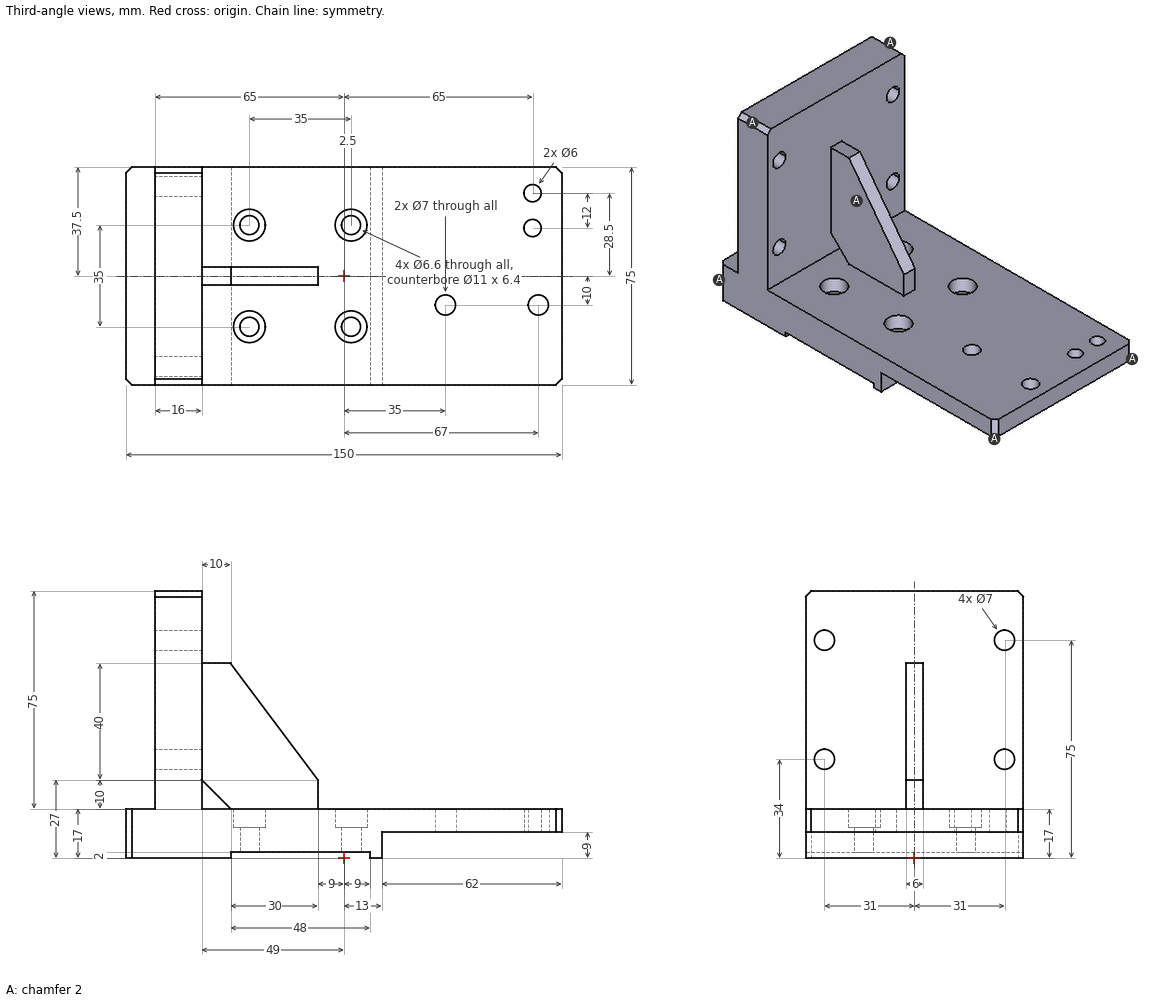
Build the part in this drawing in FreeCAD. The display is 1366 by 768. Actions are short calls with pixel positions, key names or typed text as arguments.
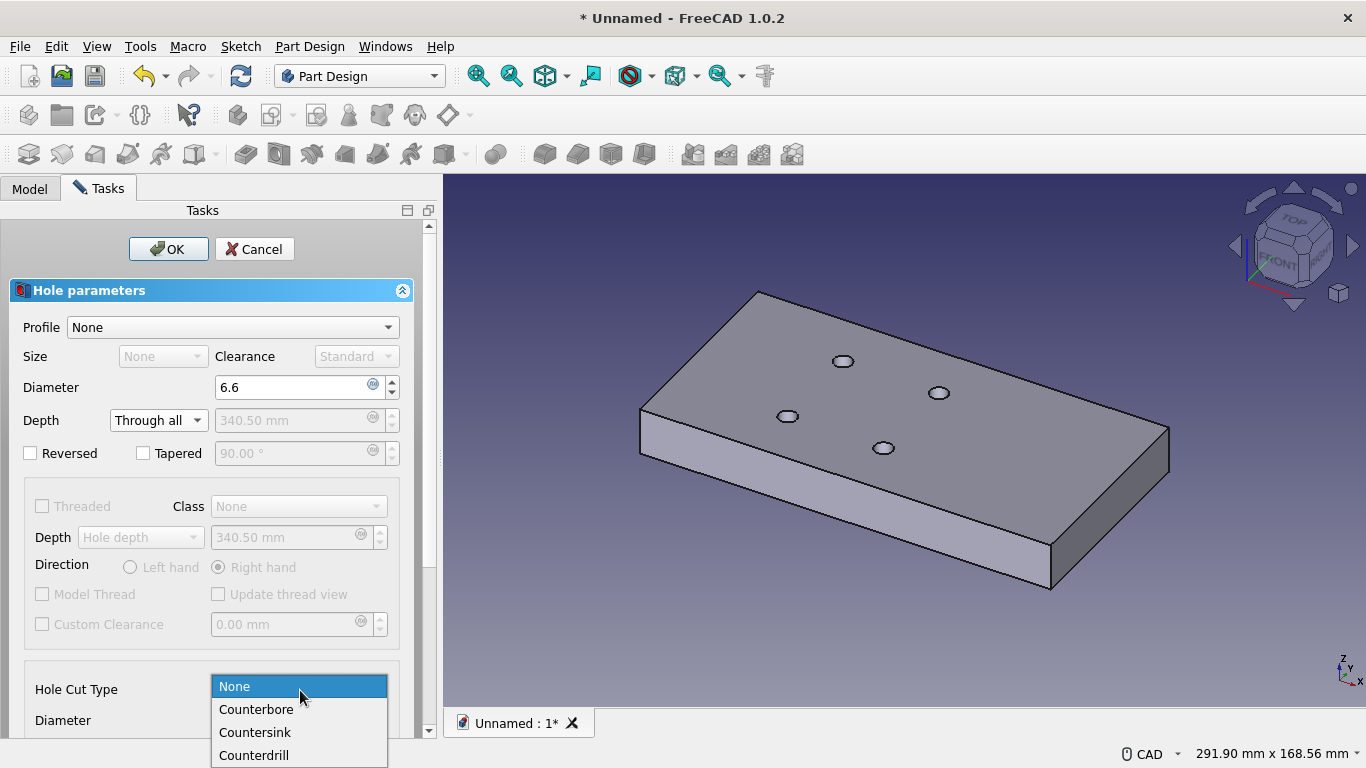
click(298, 710)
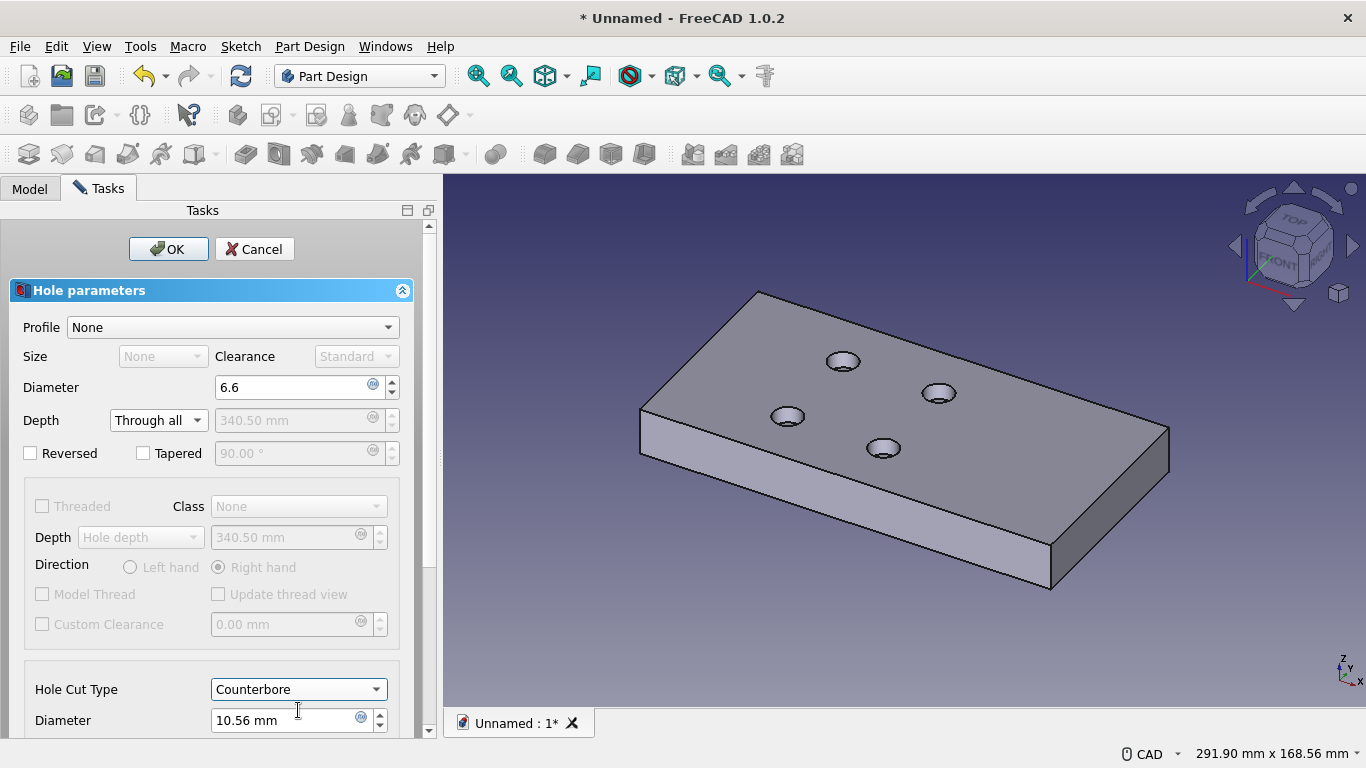
triple_click(292, 720)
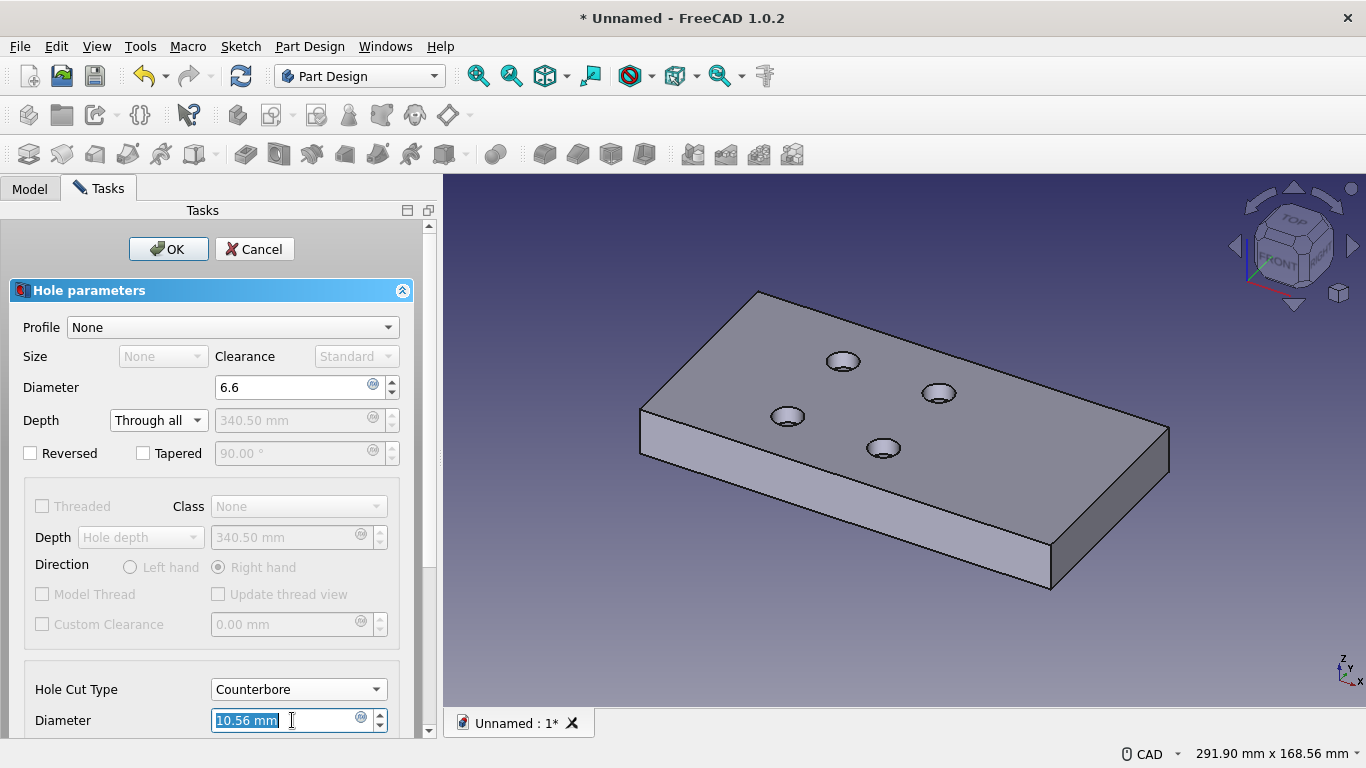
text(11)
key(Tab)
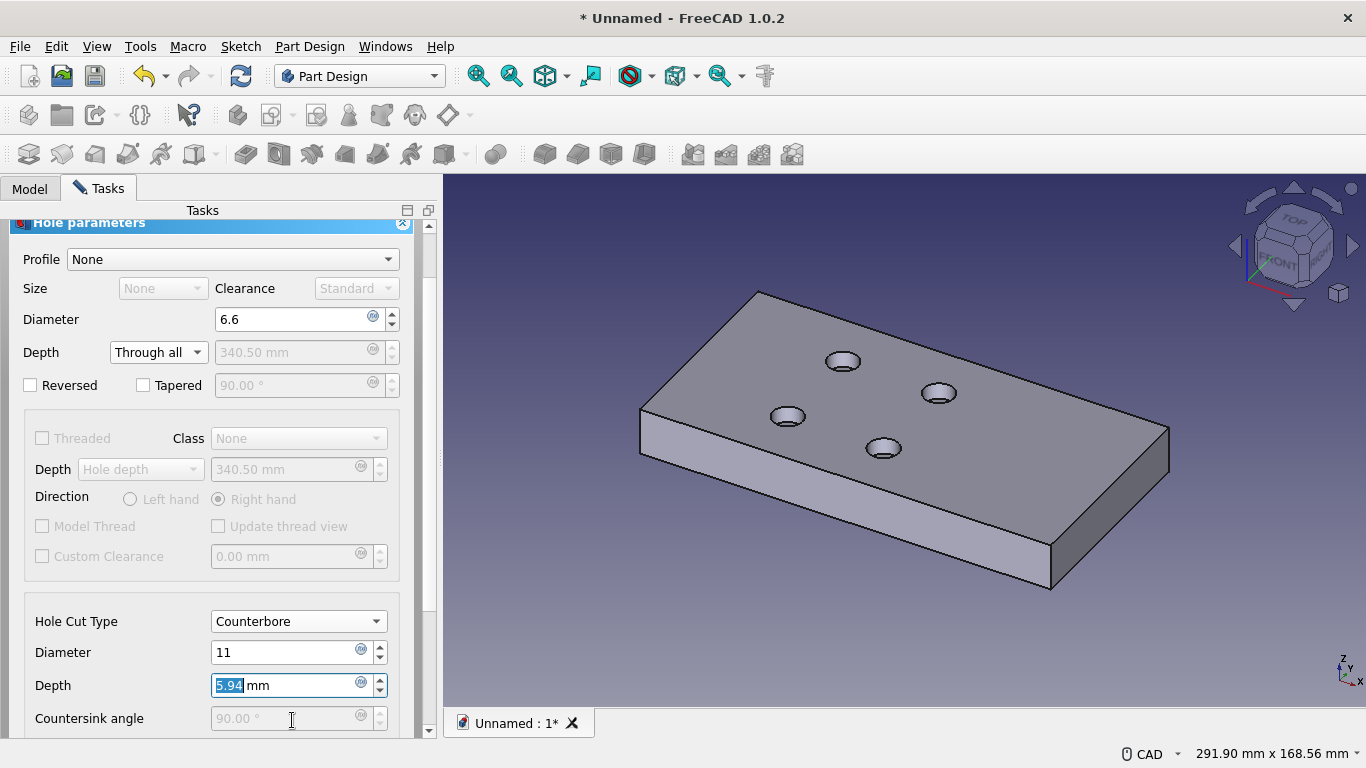
text(6.4)
key(Tab)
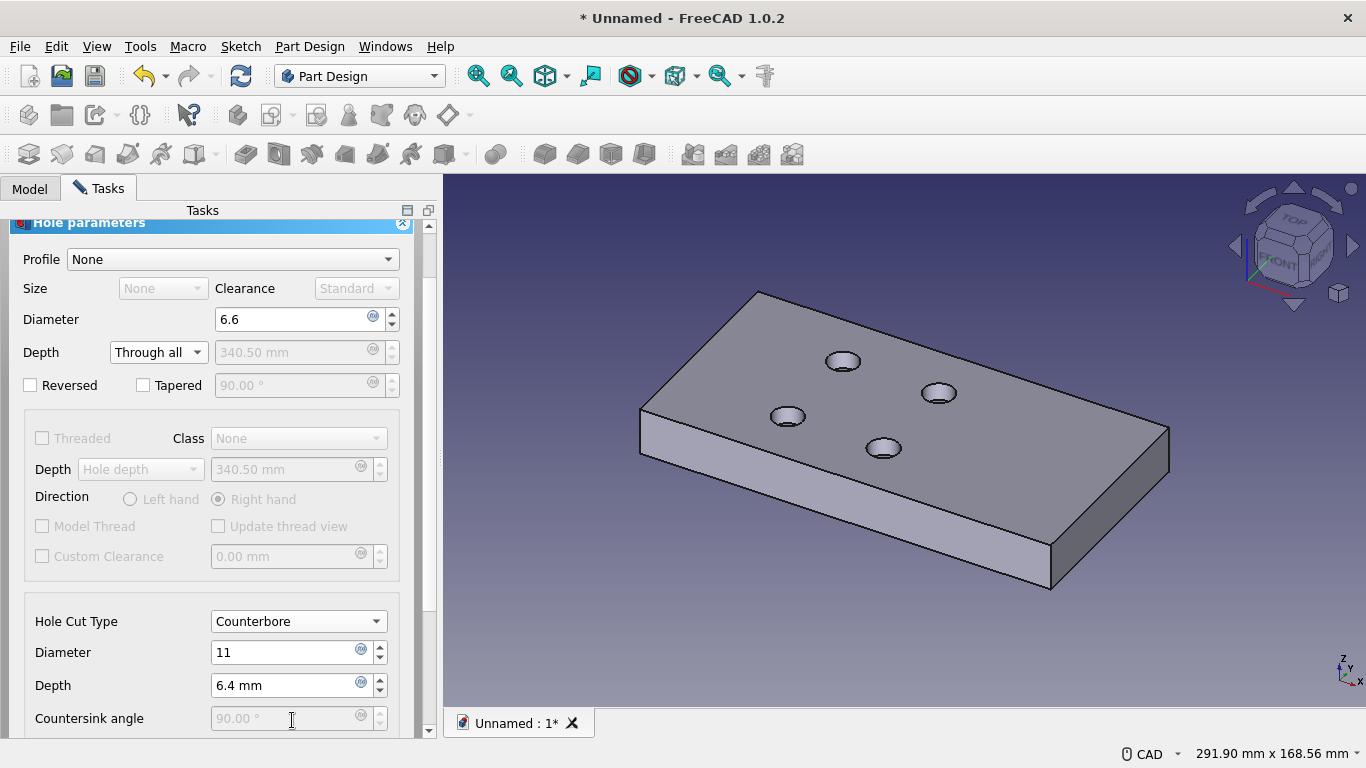
scroll(429, 479, up, 2)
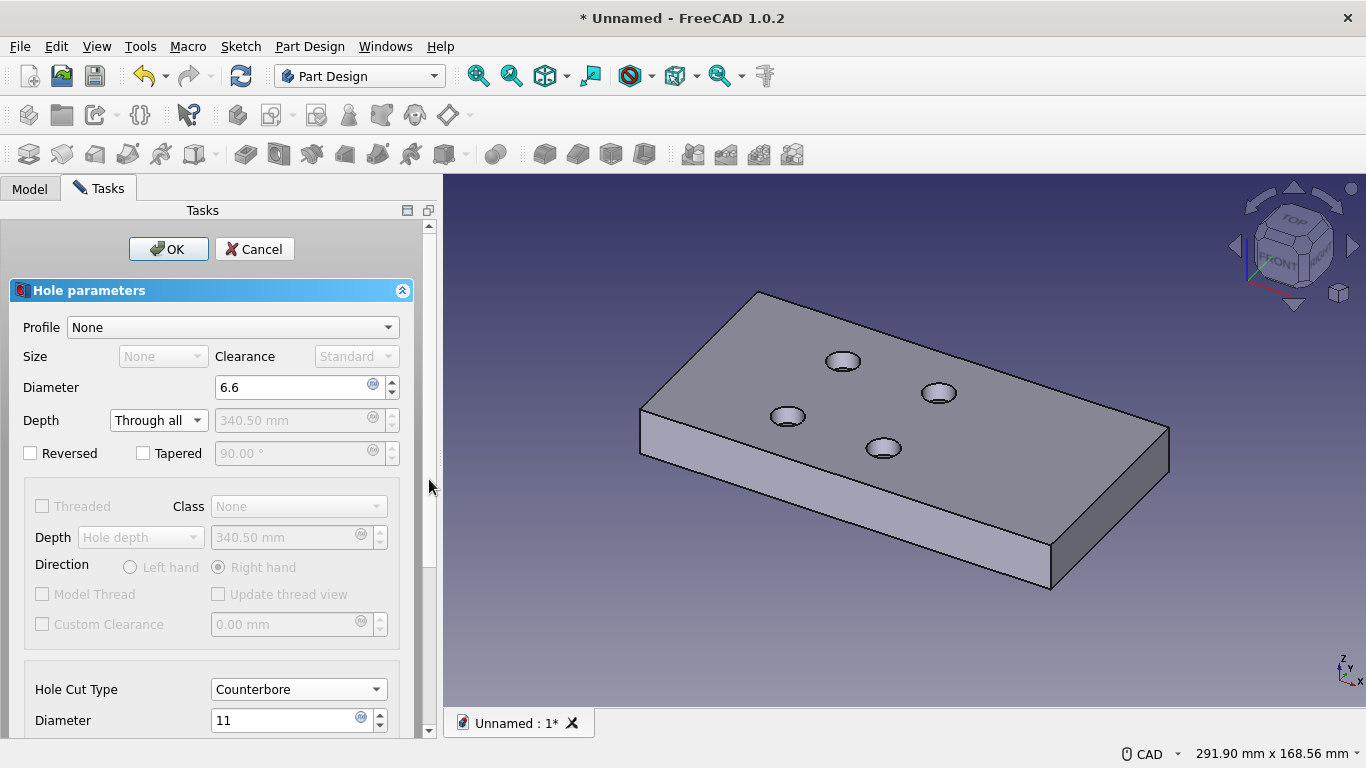
click(169, 249)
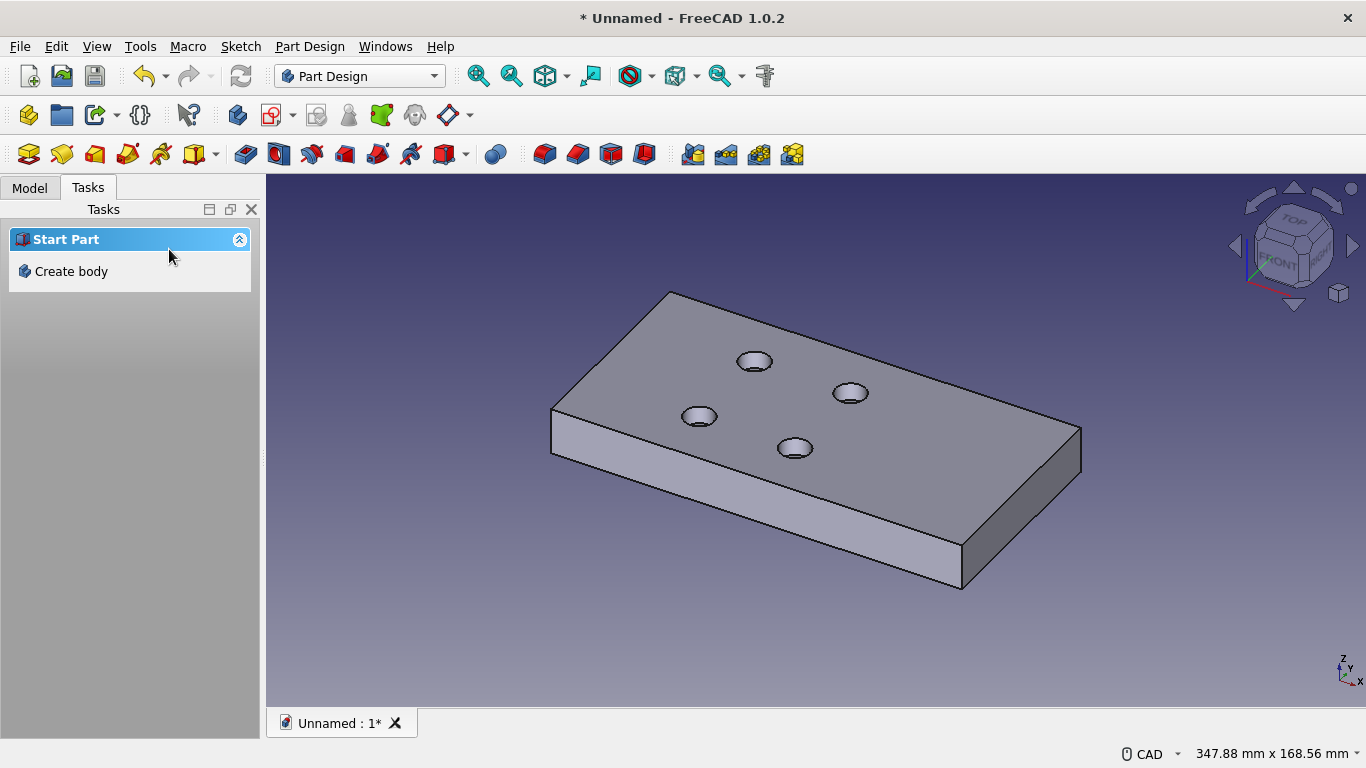
click(933, 456)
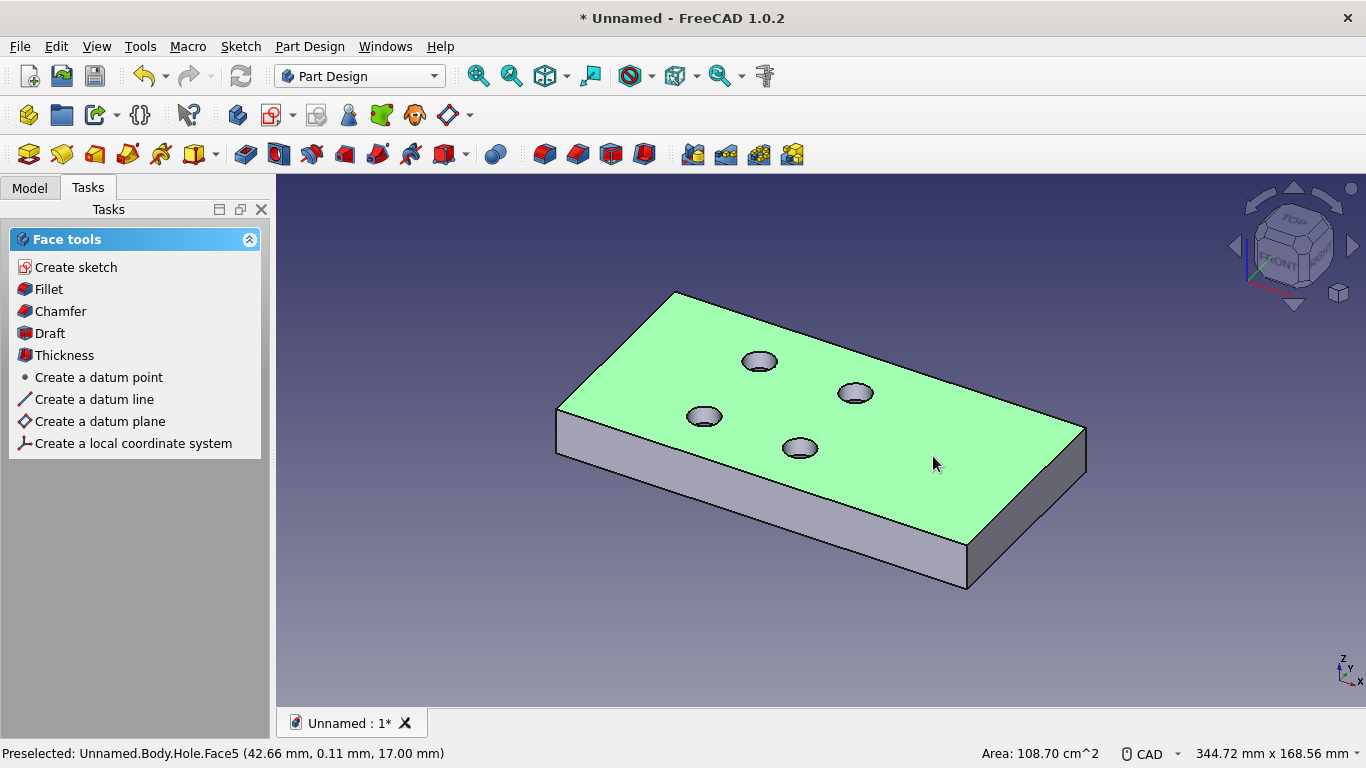
click(270, 116)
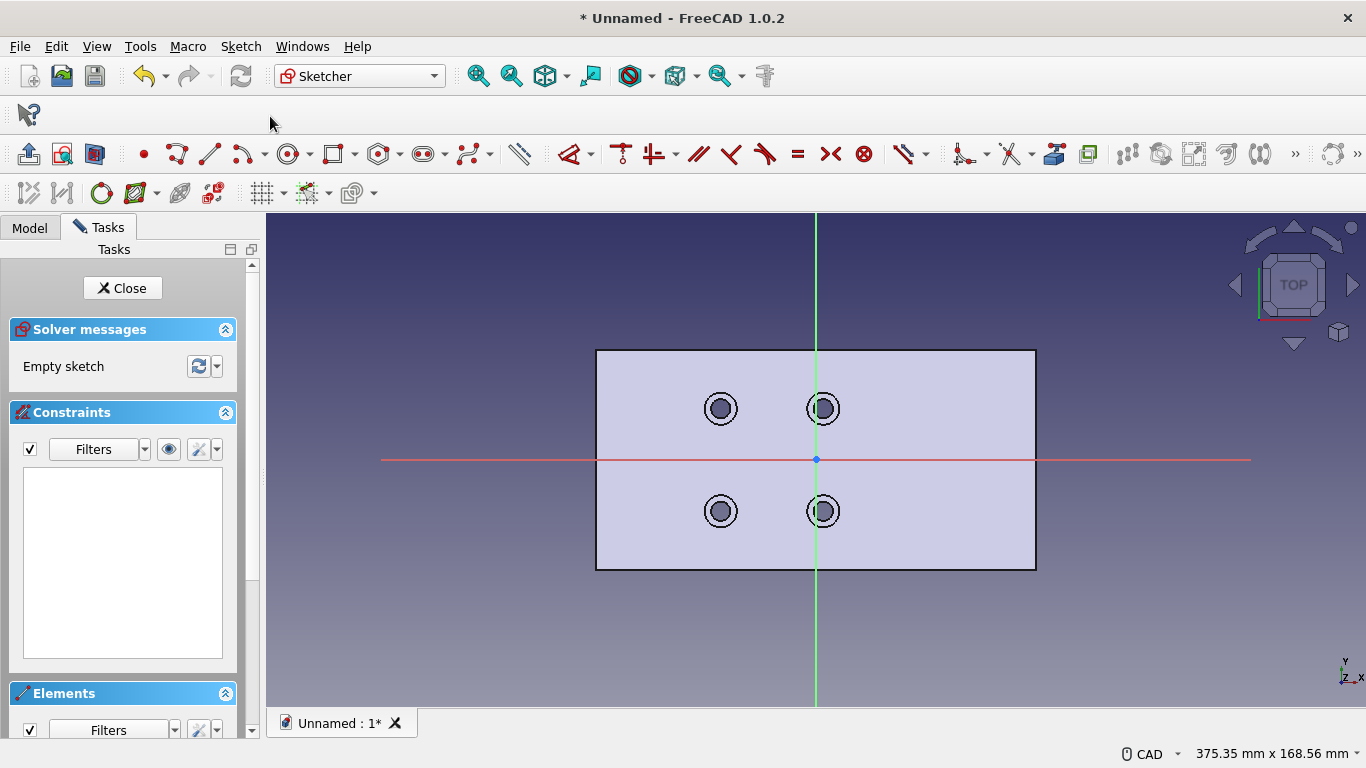
scroll(666, 460, up, 2)